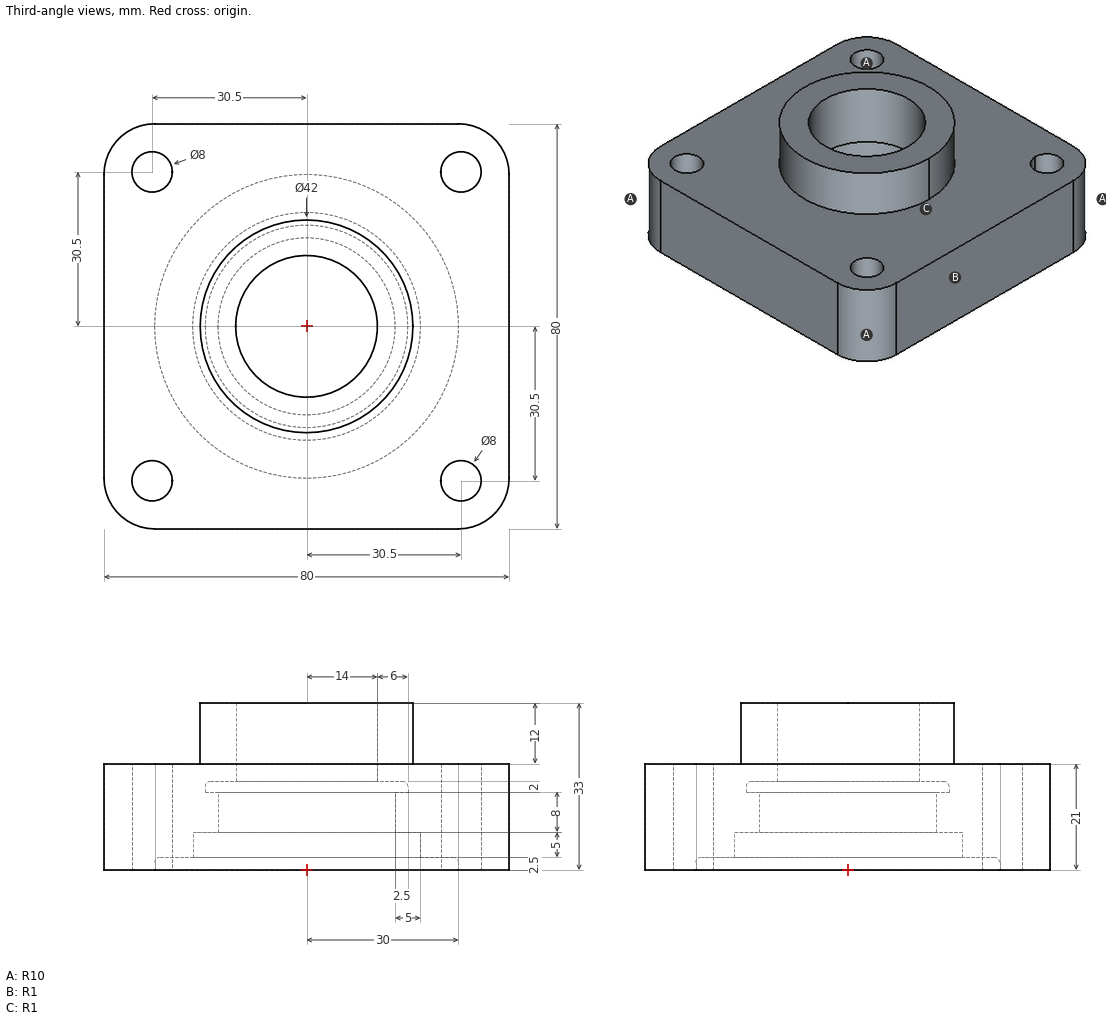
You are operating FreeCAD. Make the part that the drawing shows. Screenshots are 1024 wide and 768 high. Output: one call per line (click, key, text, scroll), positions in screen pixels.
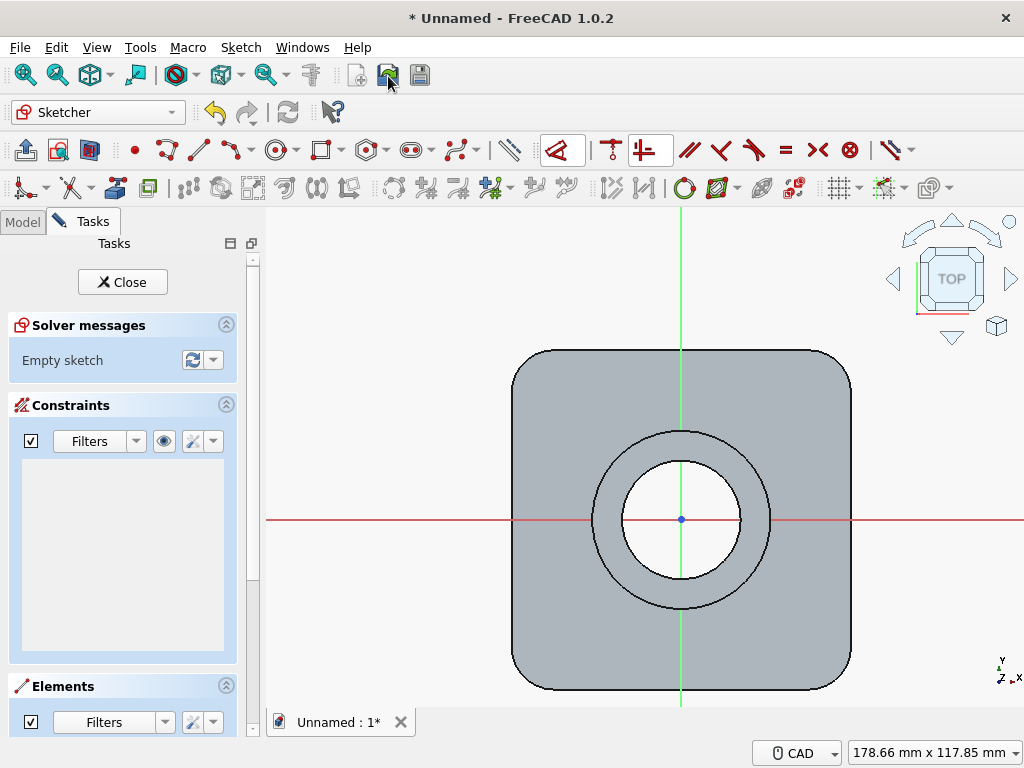
scroll(549, 382, up, 11)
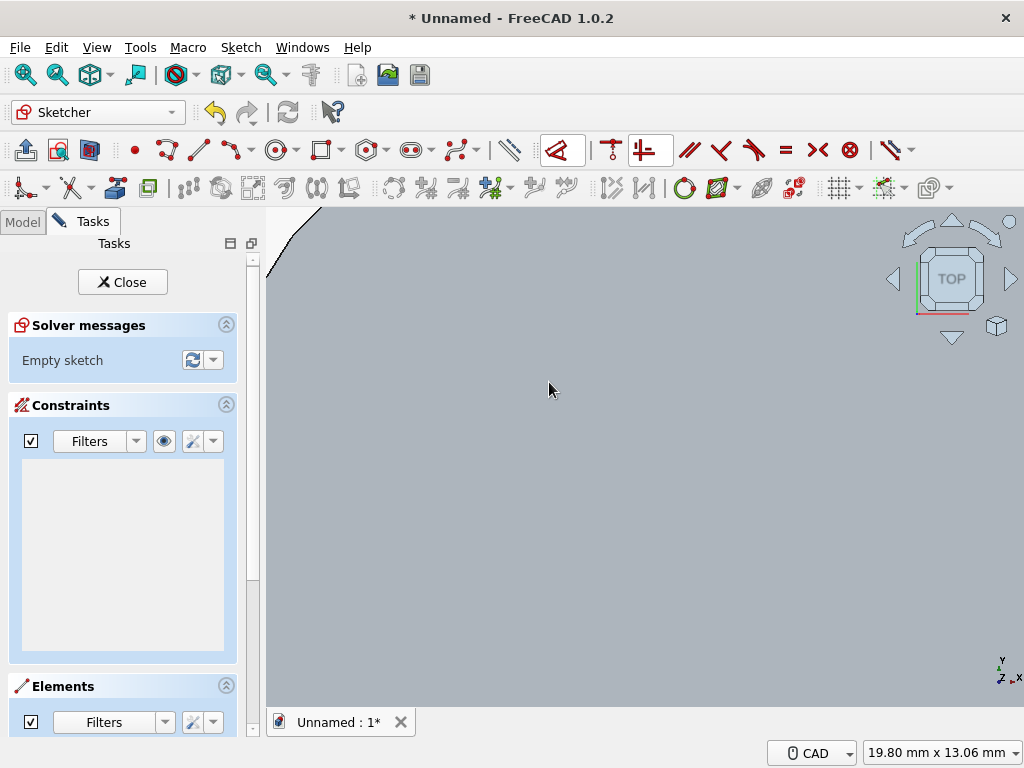
click(276, 150)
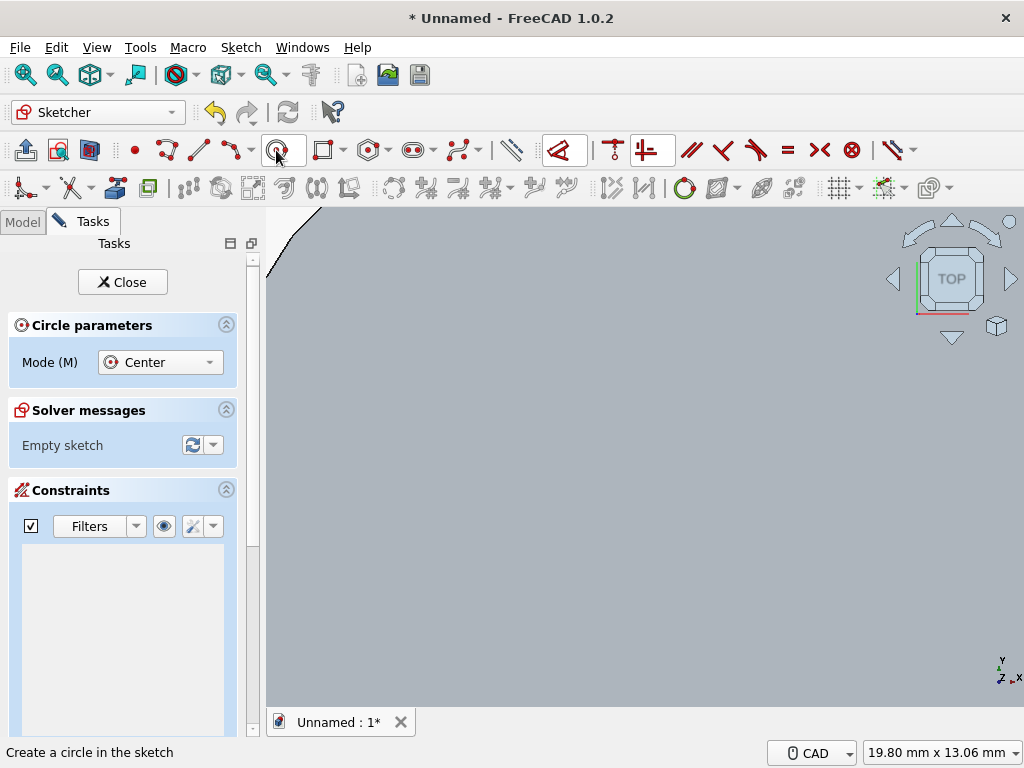
click(572, 456)
move(681, 348)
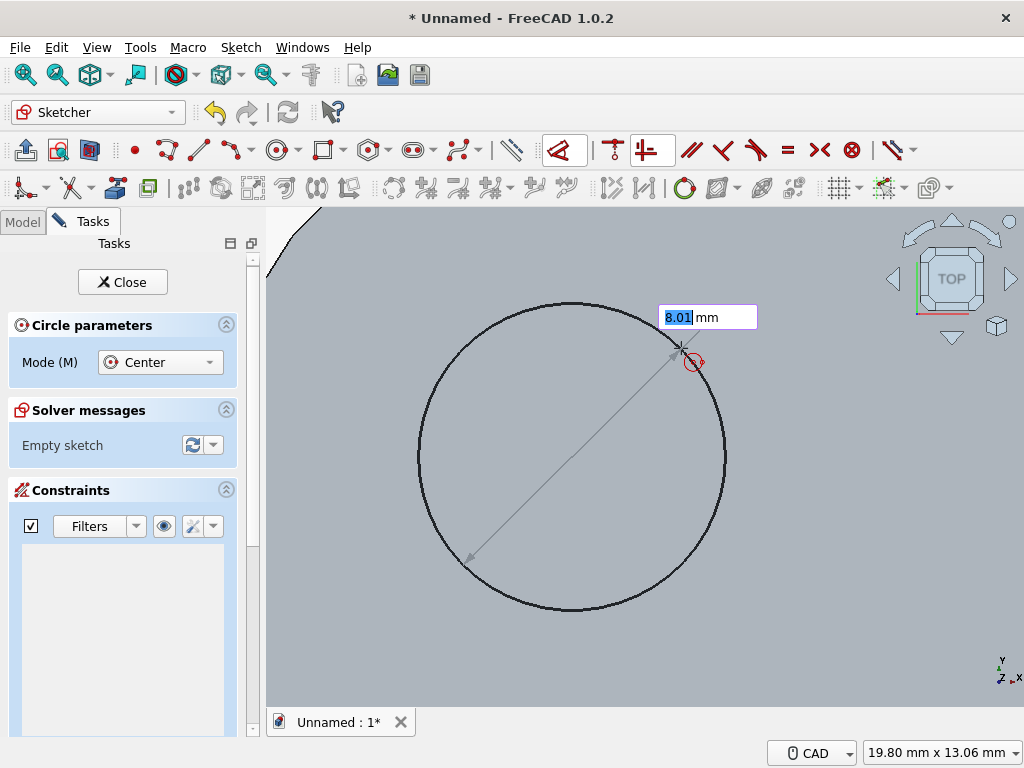
text(8)
key(Return)
key(Escape)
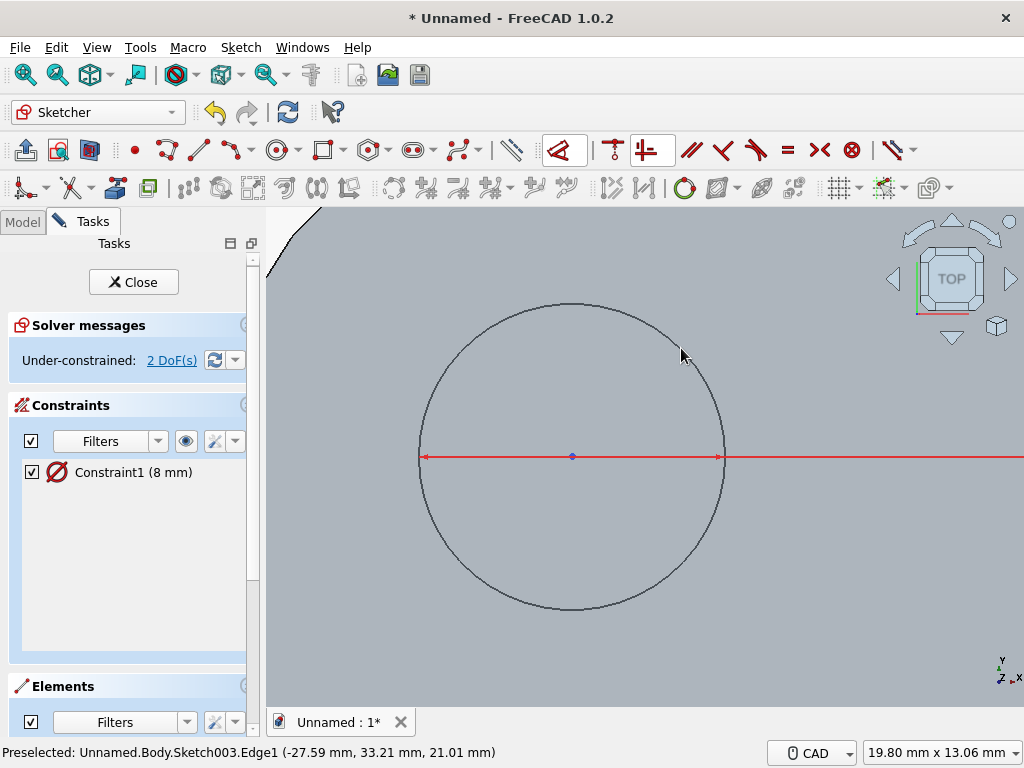
click(572, 457)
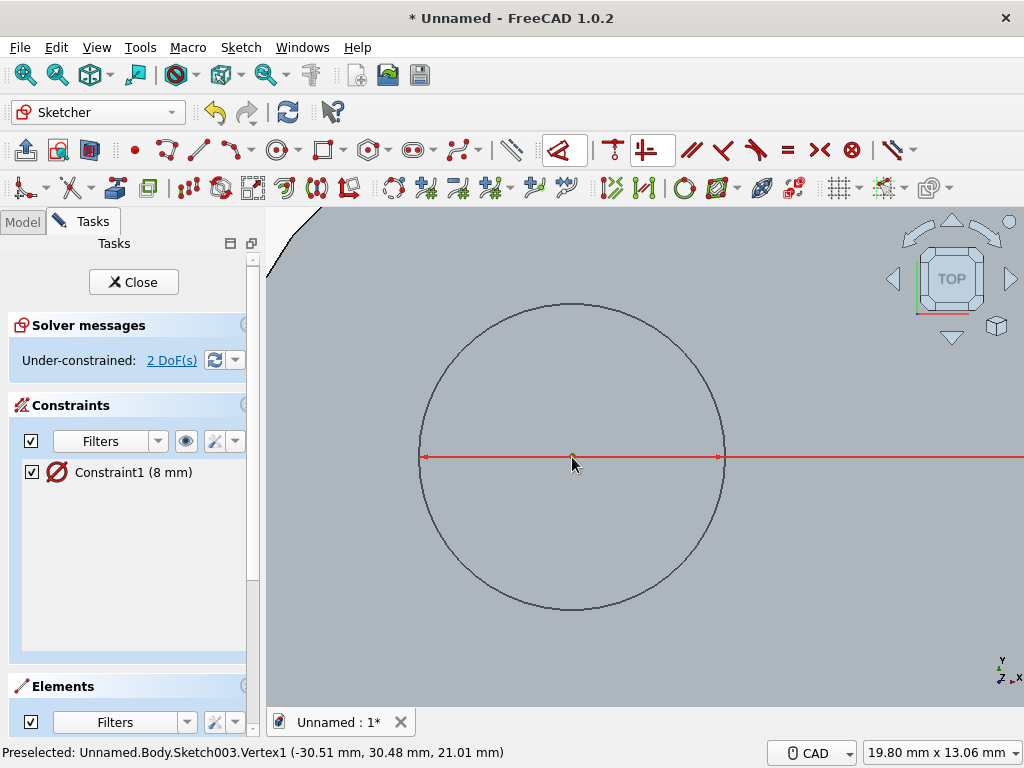
click(582, 150)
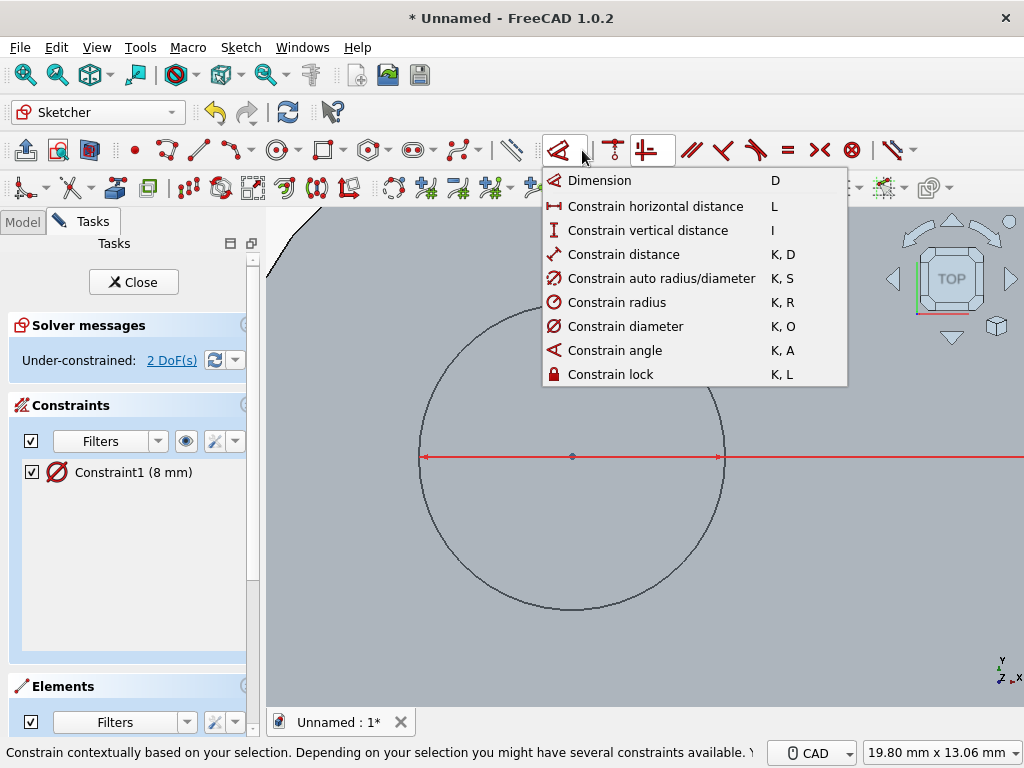
click(695, 206)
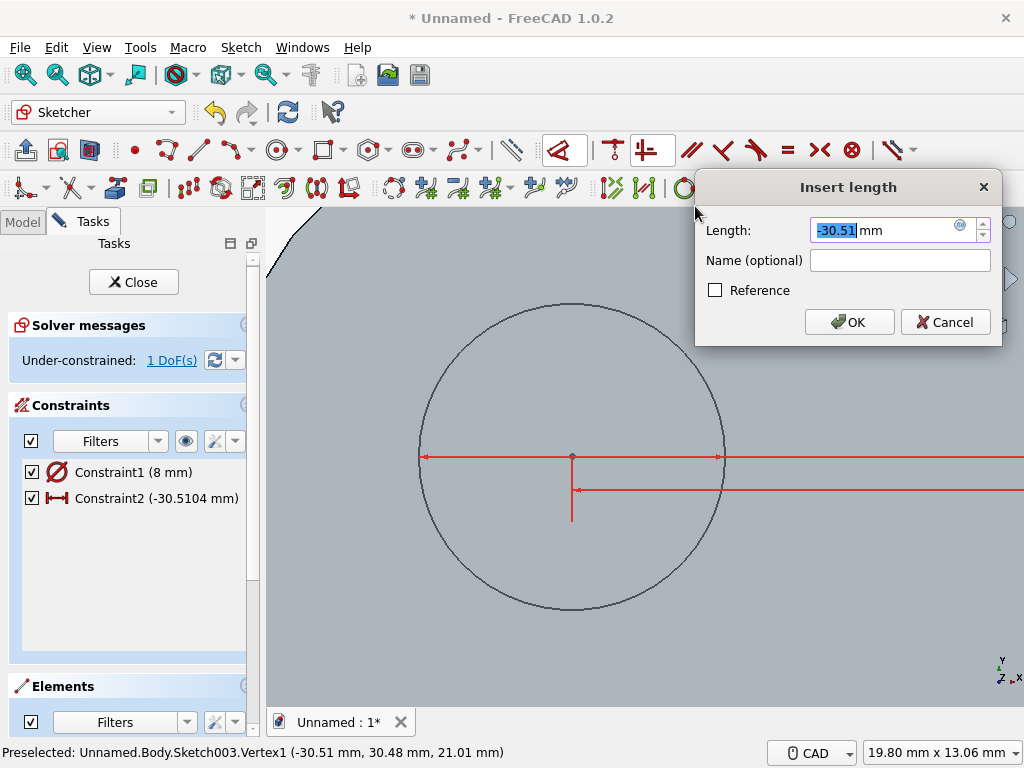
text(-30.5)
key(Return)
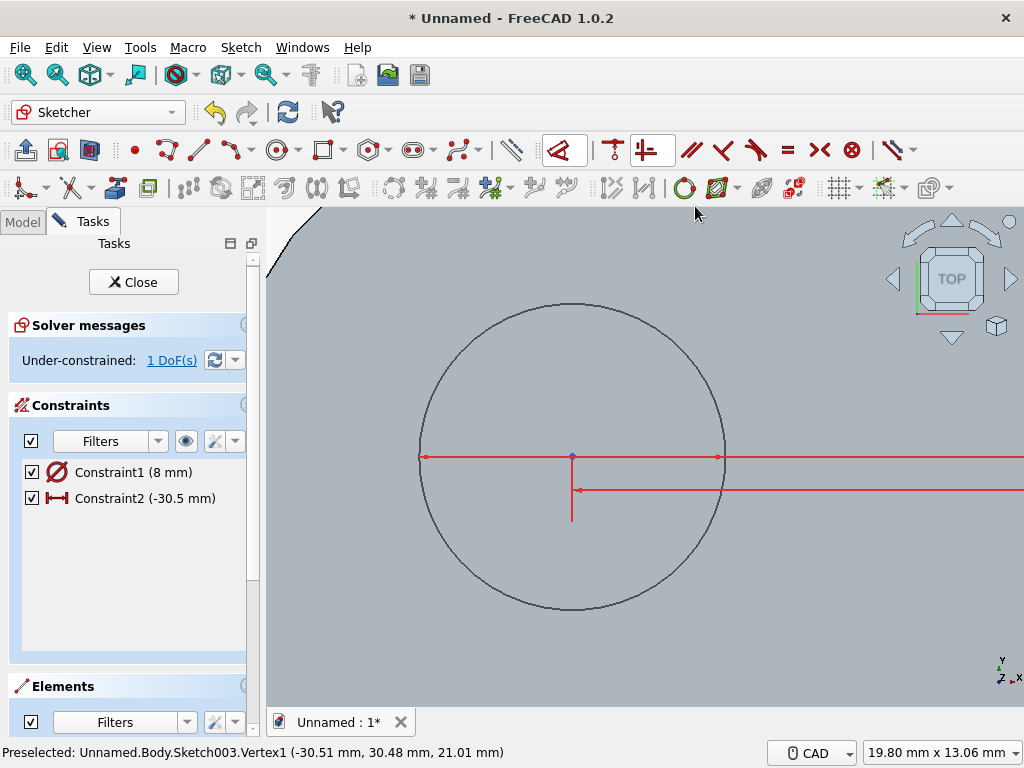
click(572, 457)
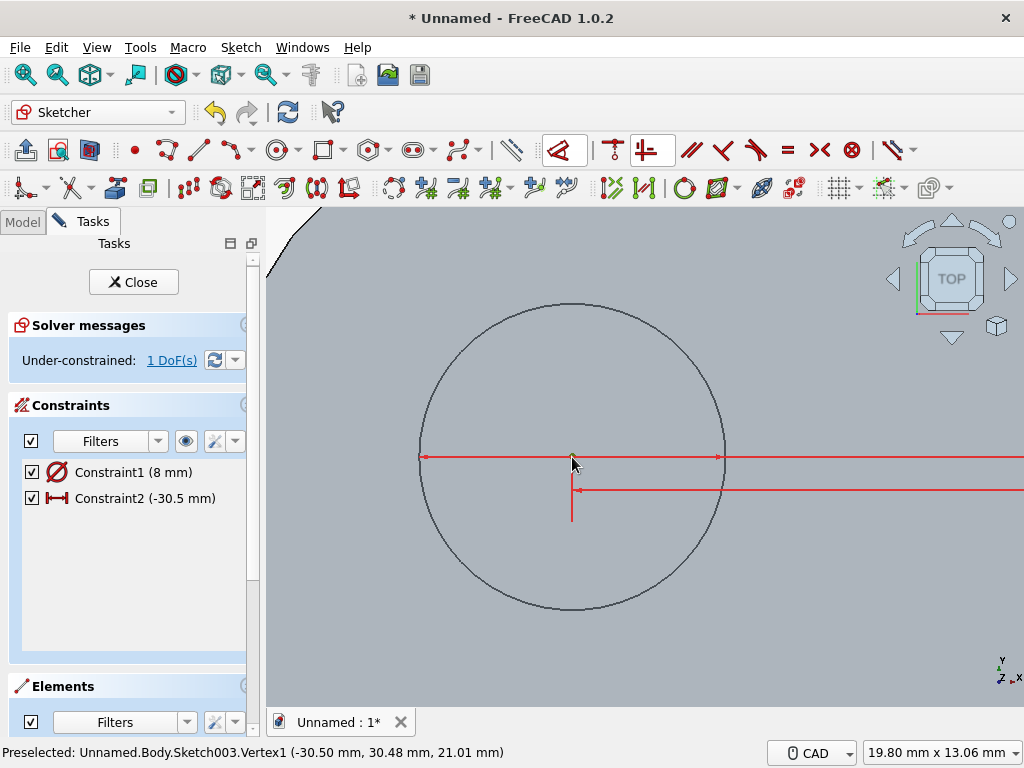
key(i)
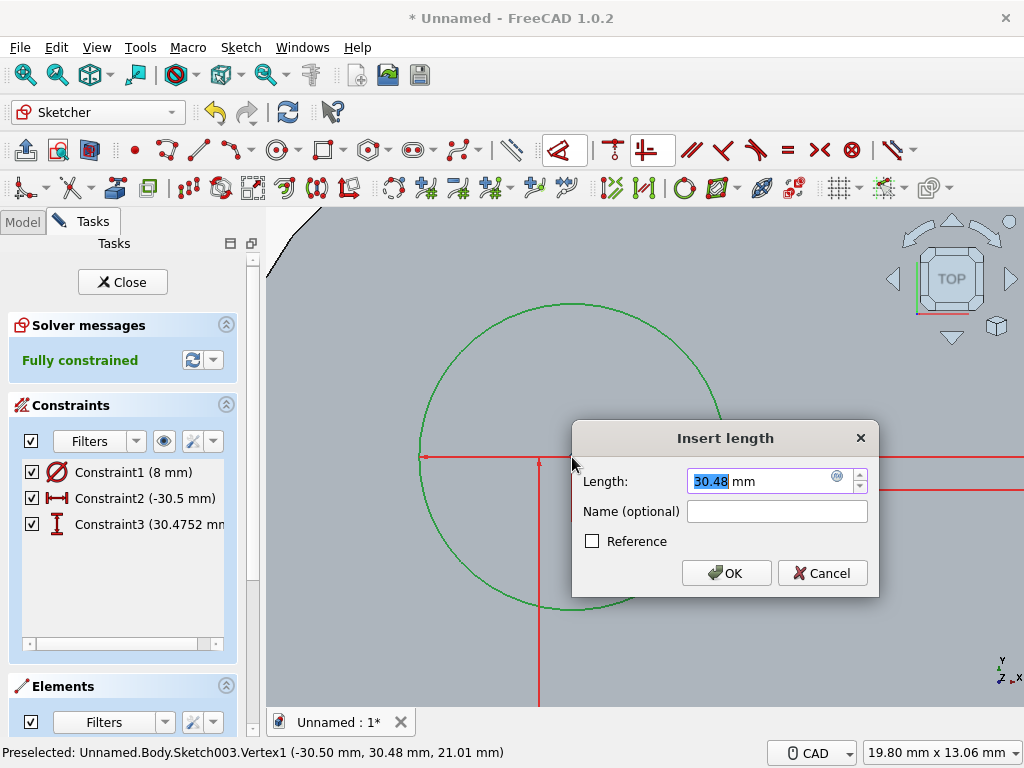
text(30.5)
key(Return)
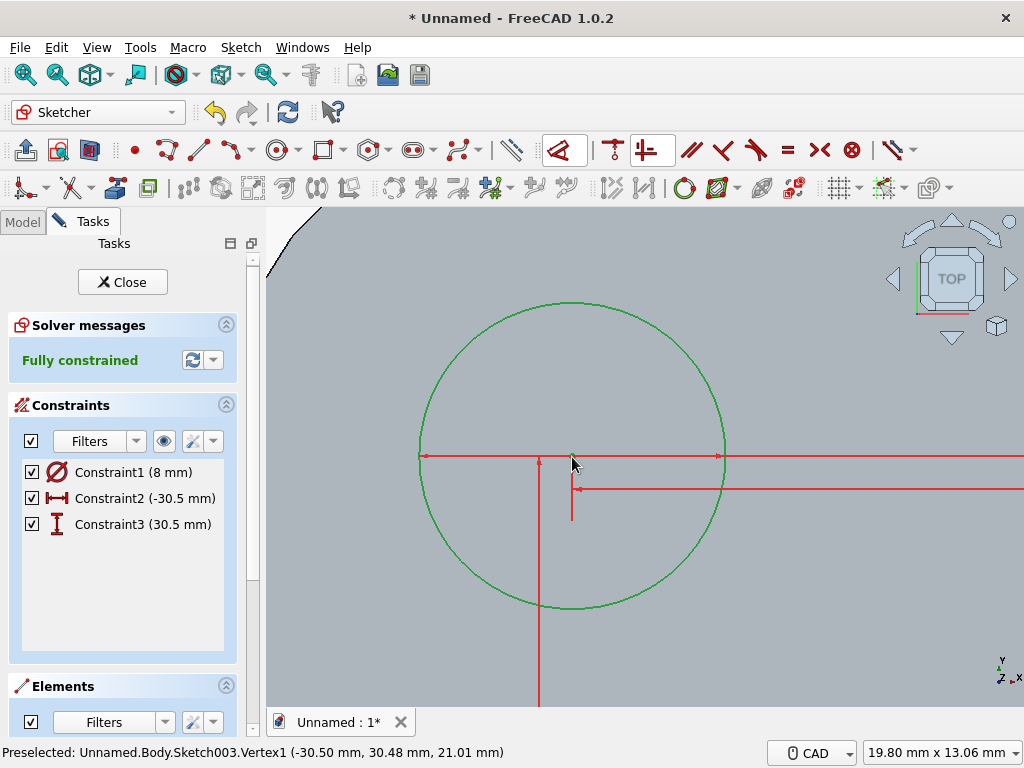
click(123, 282)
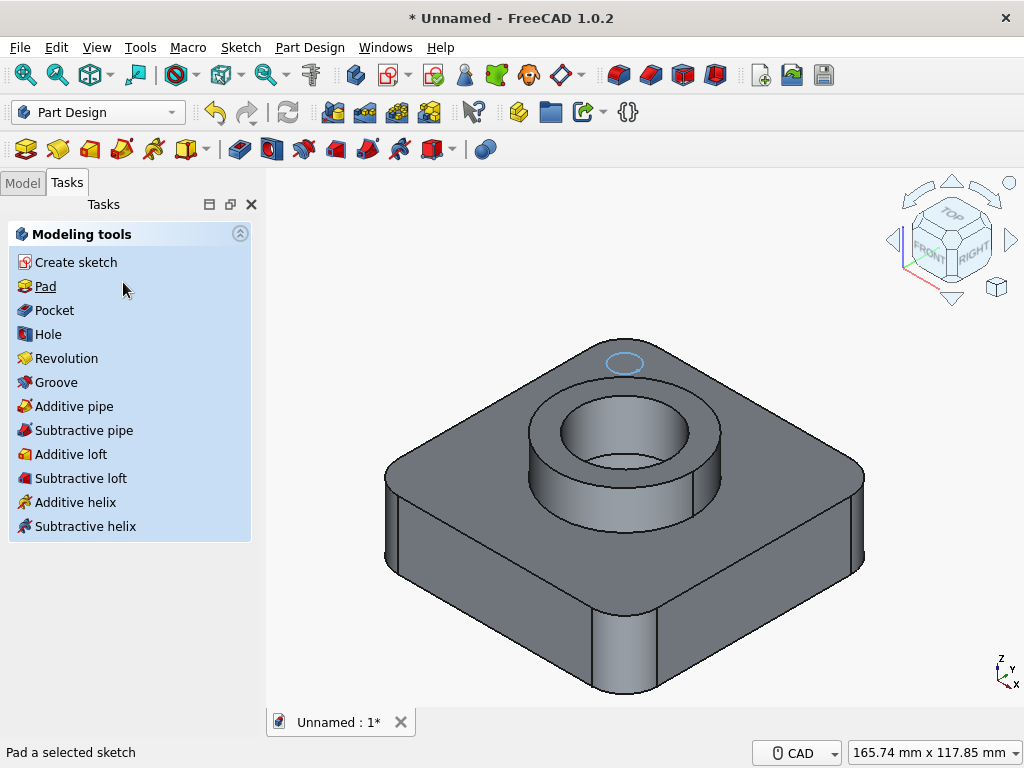
click(240, 150)